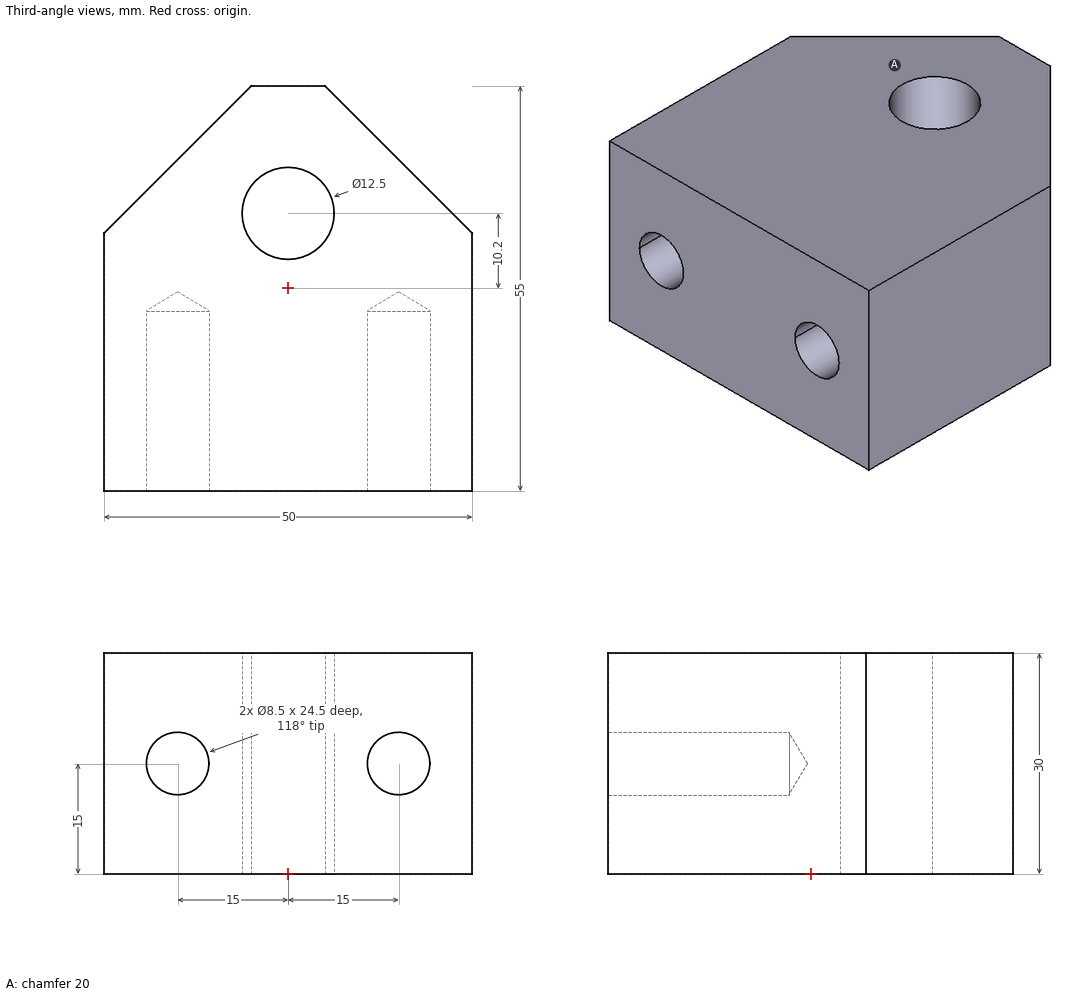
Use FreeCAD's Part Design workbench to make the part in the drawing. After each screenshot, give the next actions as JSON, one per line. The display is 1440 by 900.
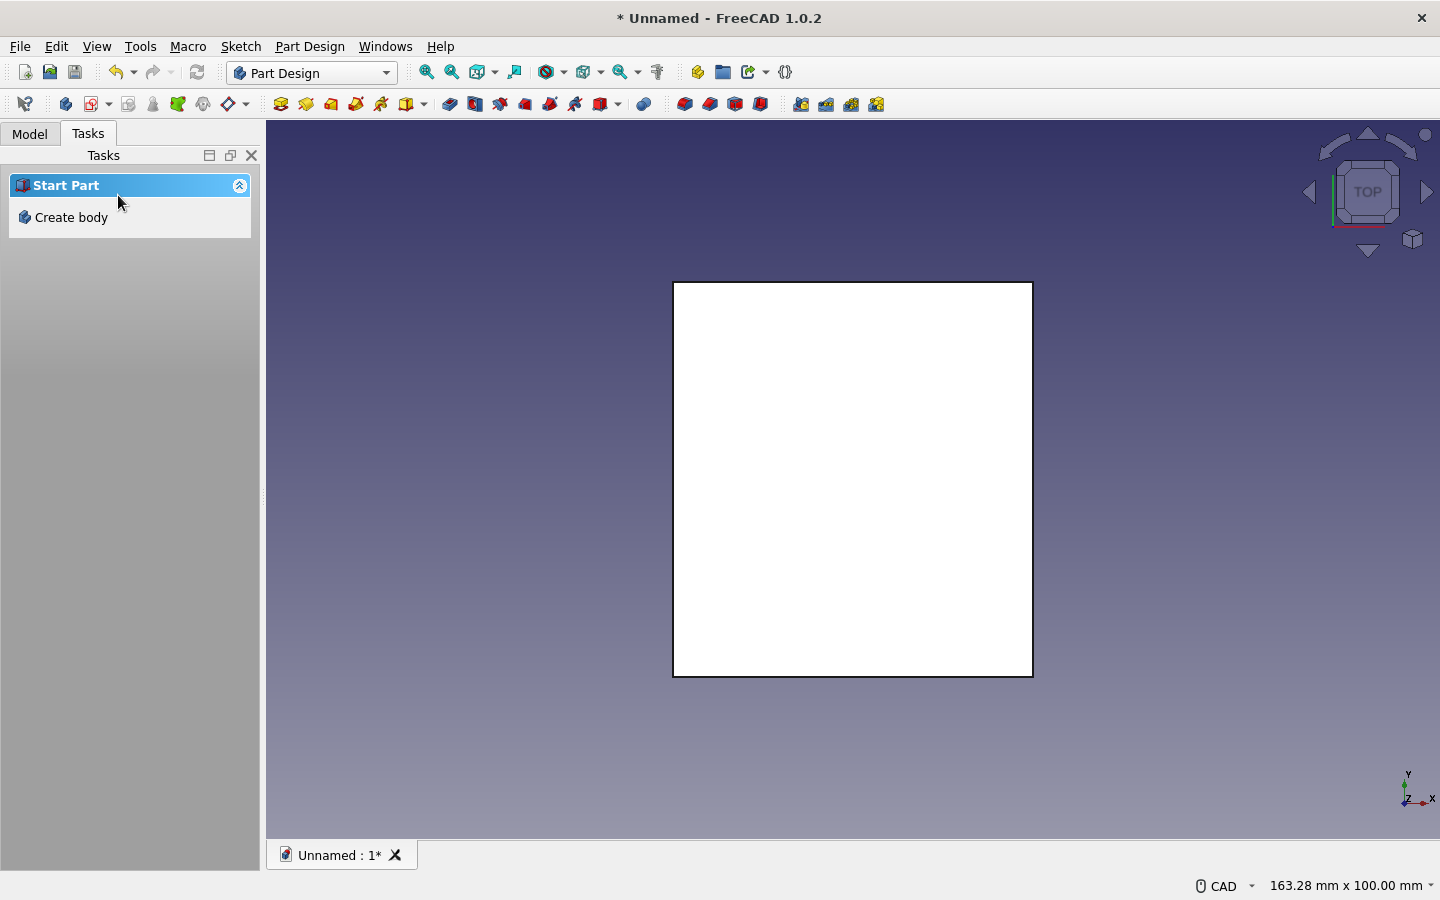
{"action": "key", "text": "1"}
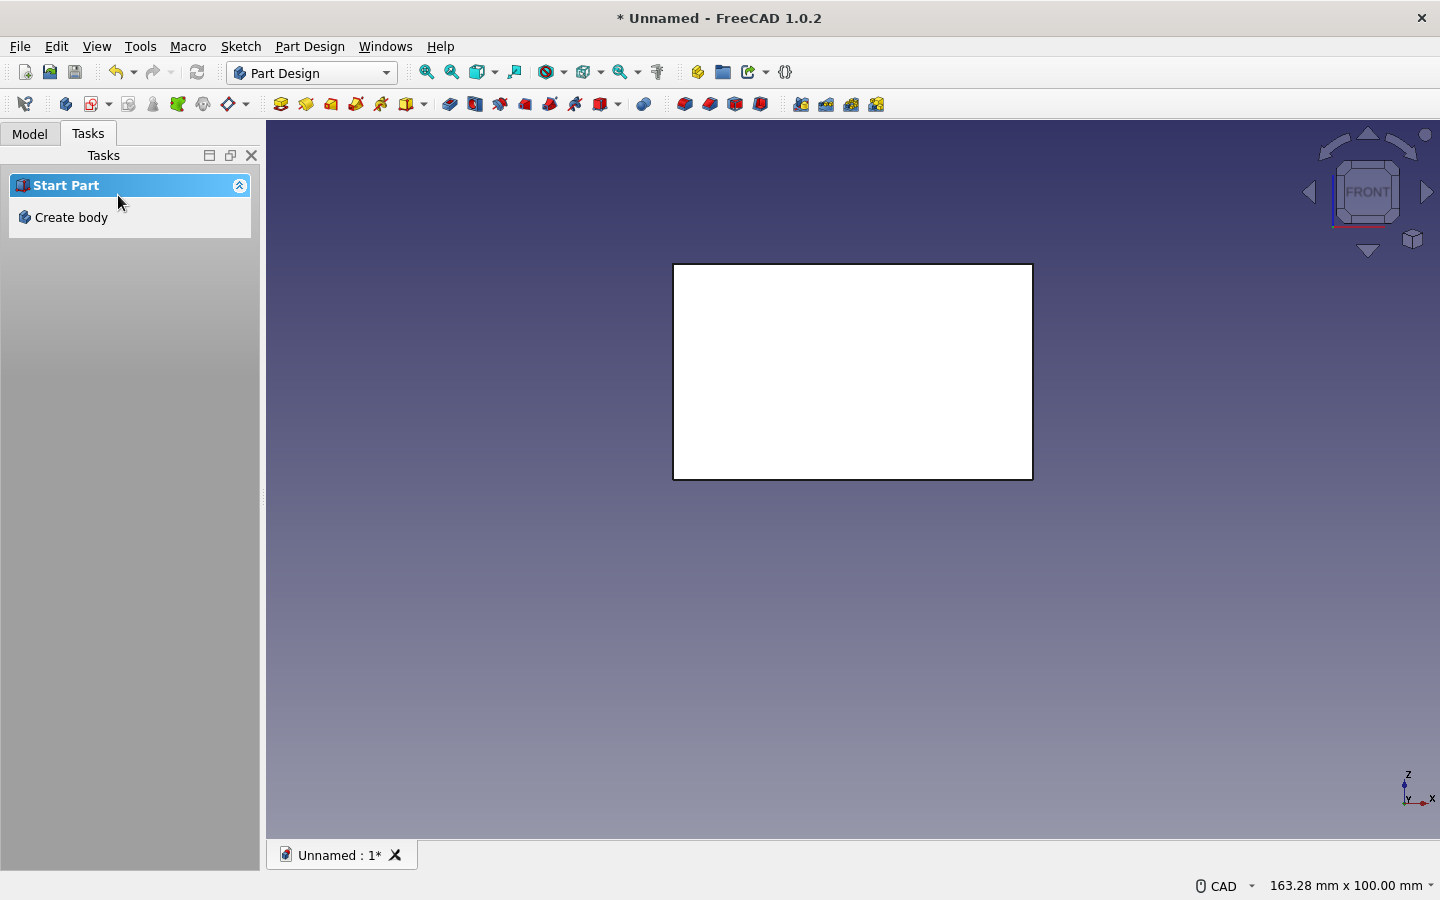
{"action": "left_click", "coordinate": [427, 72]}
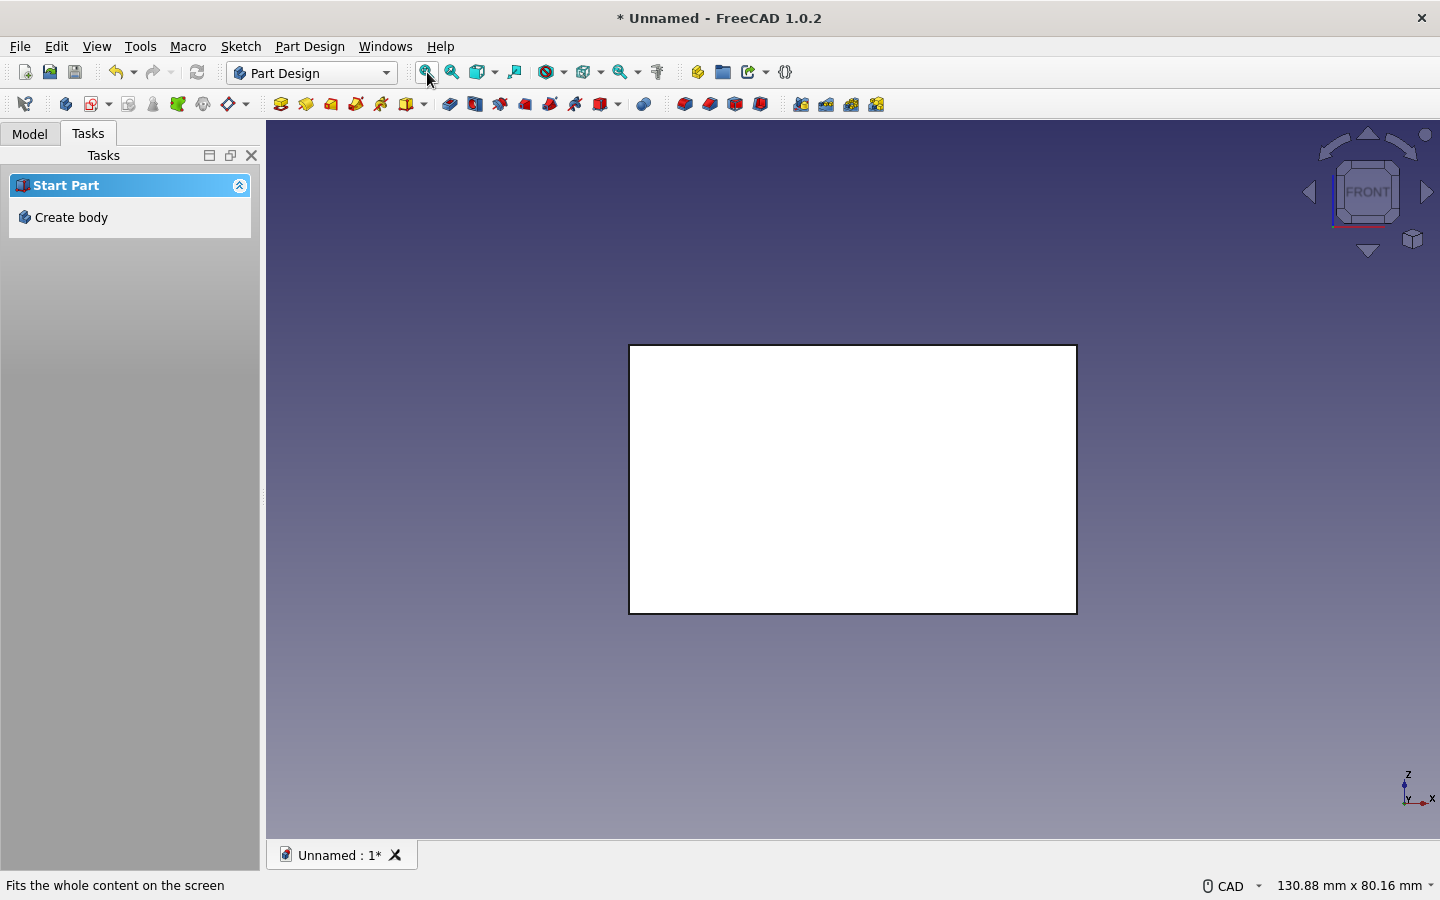
{"action": "key", "text": "3"}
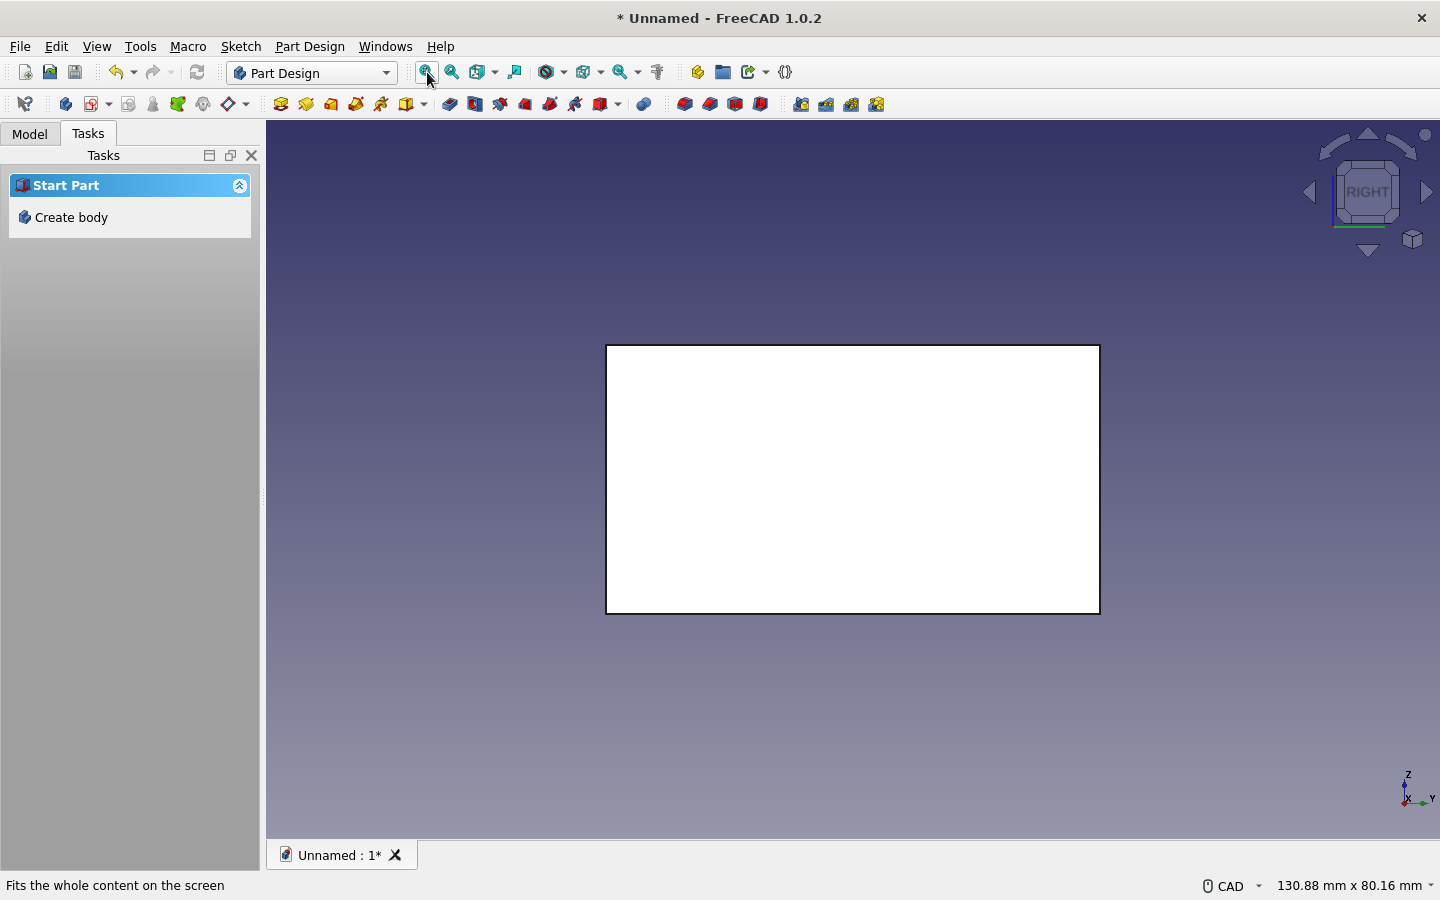
{"action": "left_click", "coordinate": [427, 72]}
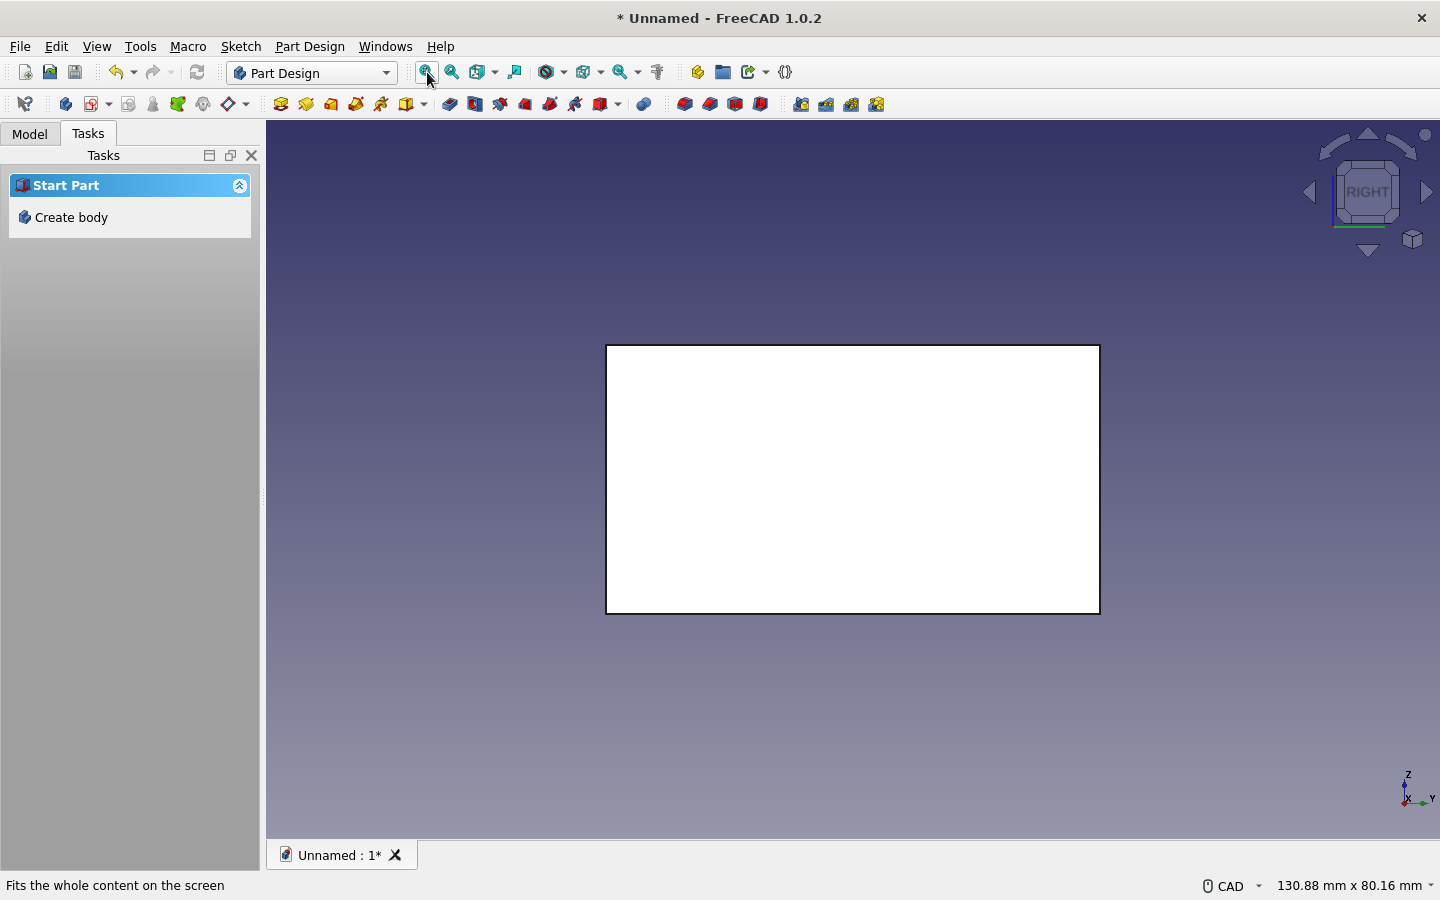
{"action": "left_click", "coordinate": [1100, 478]}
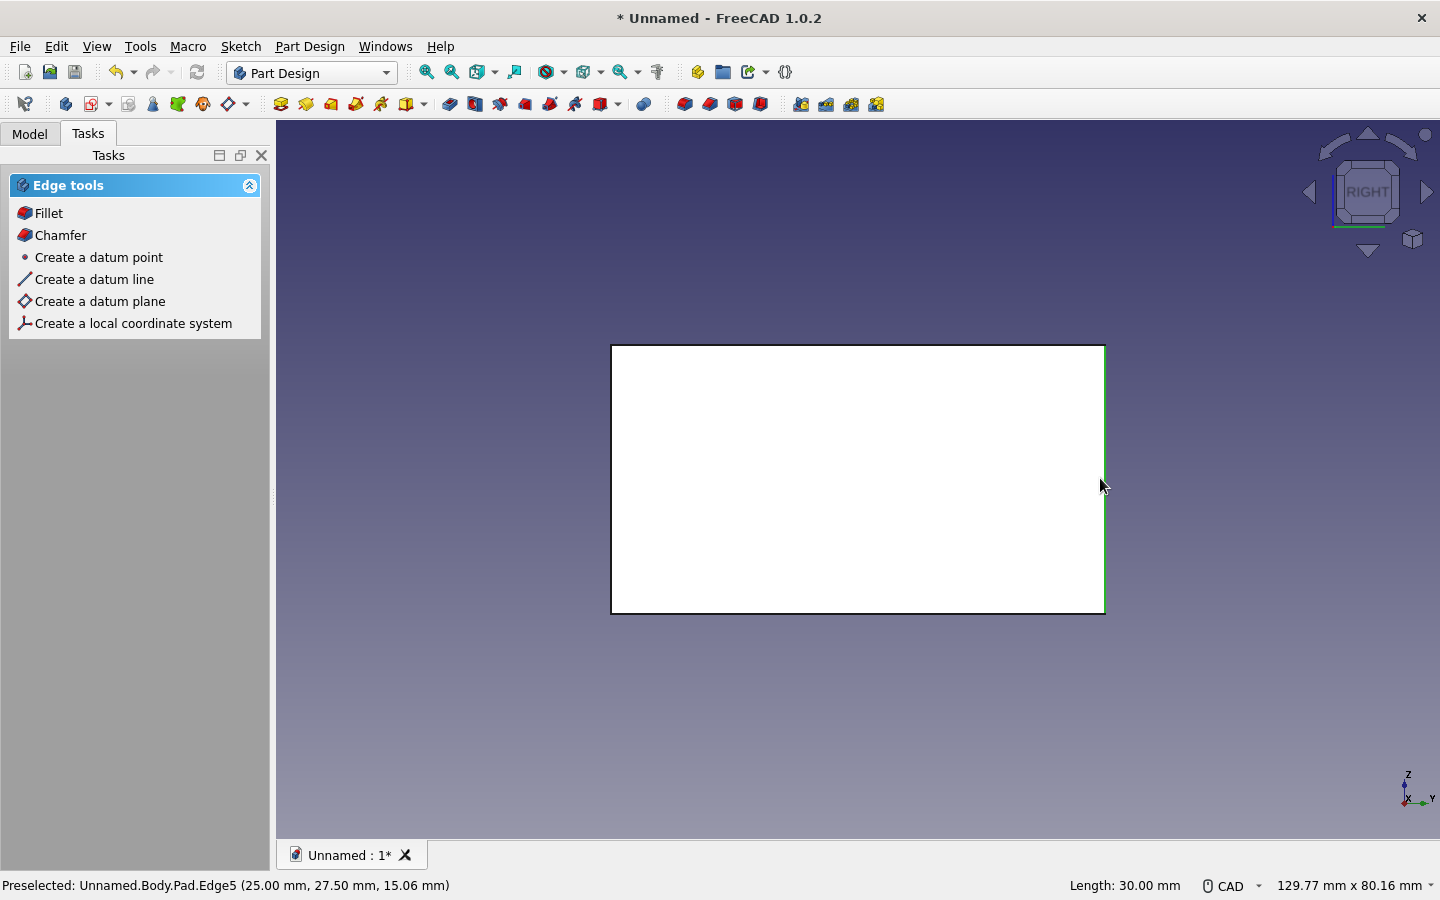
{"action": "key", "text": "5"}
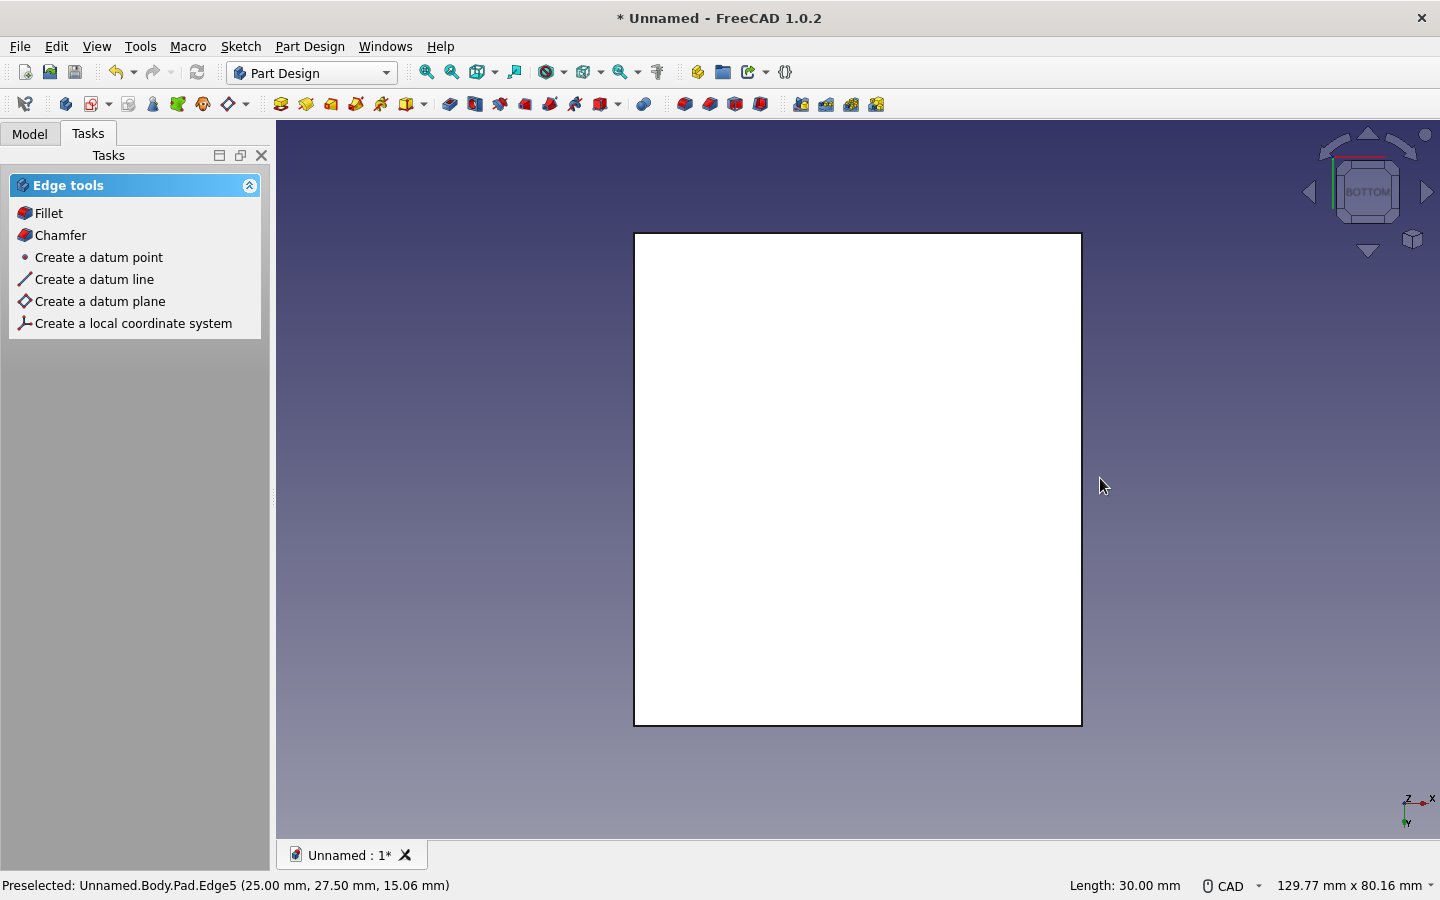
{"action": "key", "text": "4"}